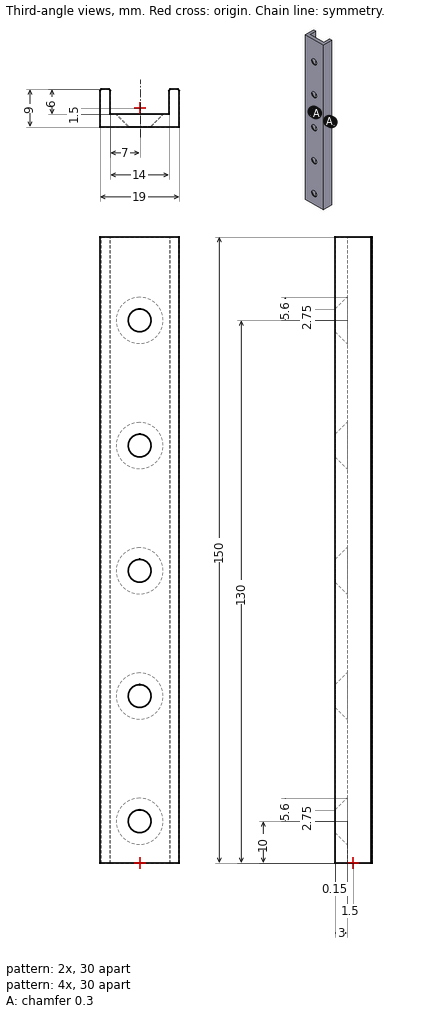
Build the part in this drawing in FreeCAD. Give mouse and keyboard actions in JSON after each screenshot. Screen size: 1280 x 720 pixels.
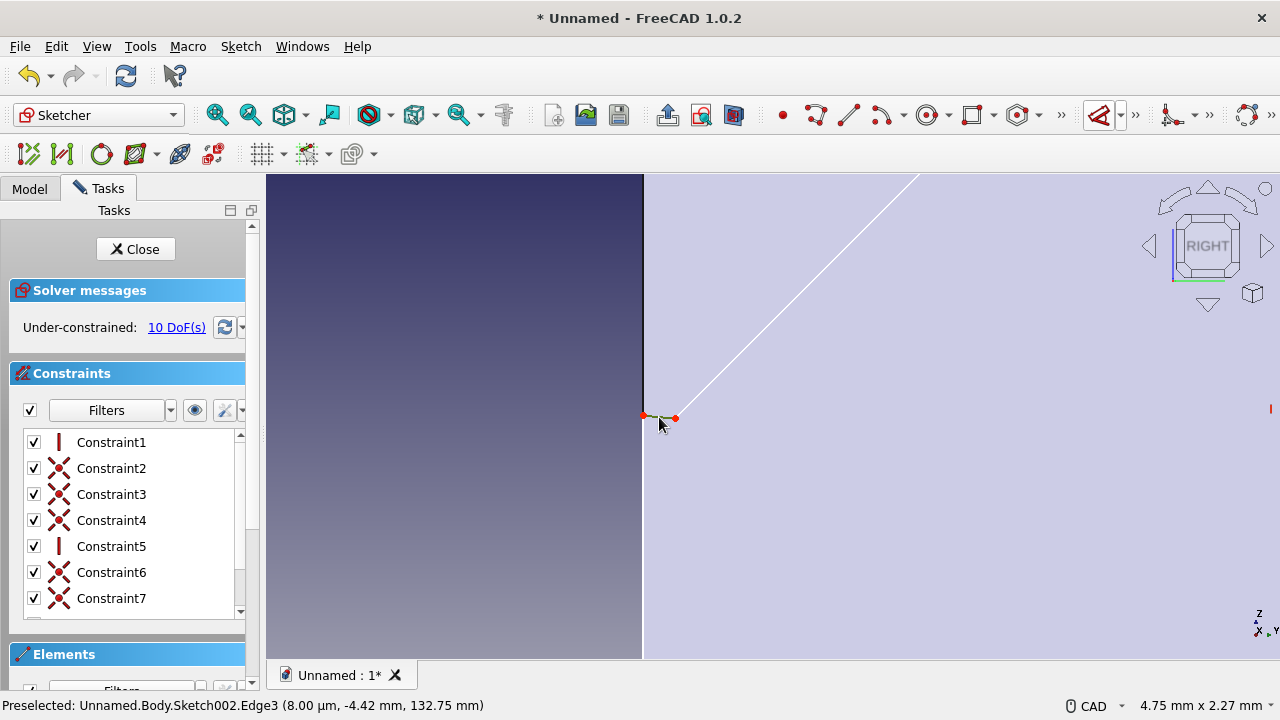
{"action": "key", "text": "h"}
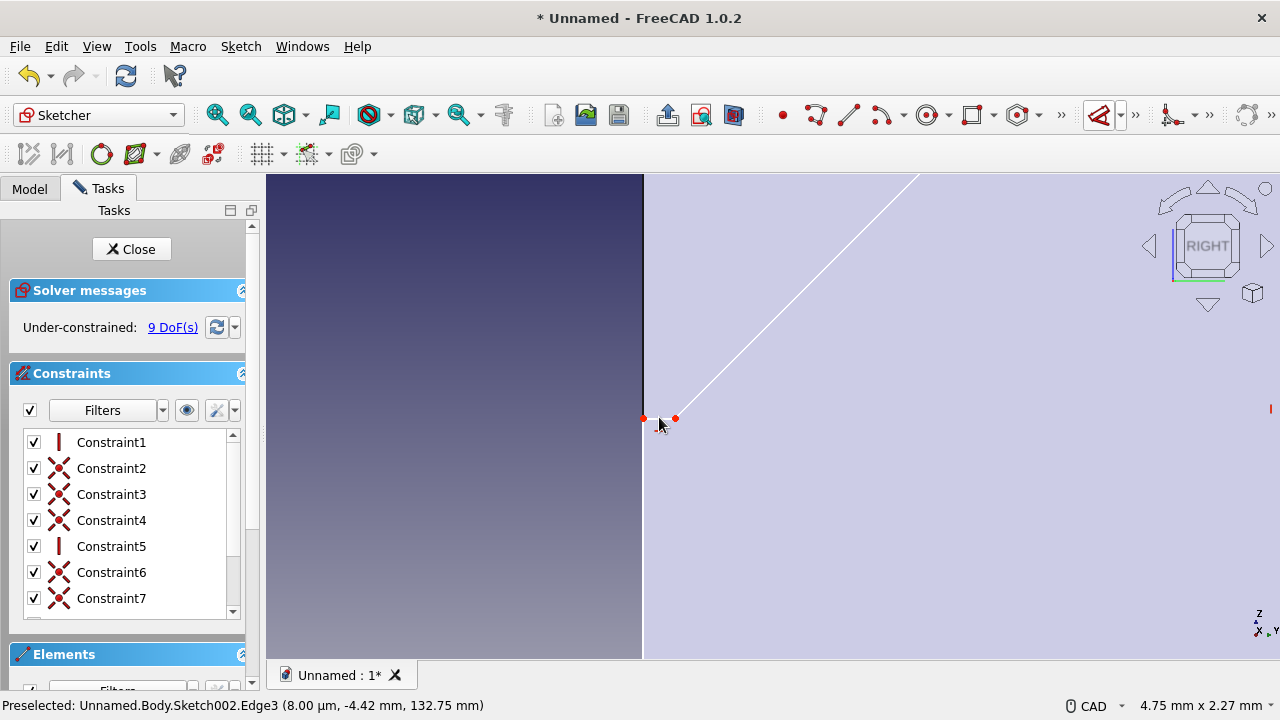
{"action": "scroll", "coordinate": [662, 420], "scroll_direction": "down", "scroll_amount": 7}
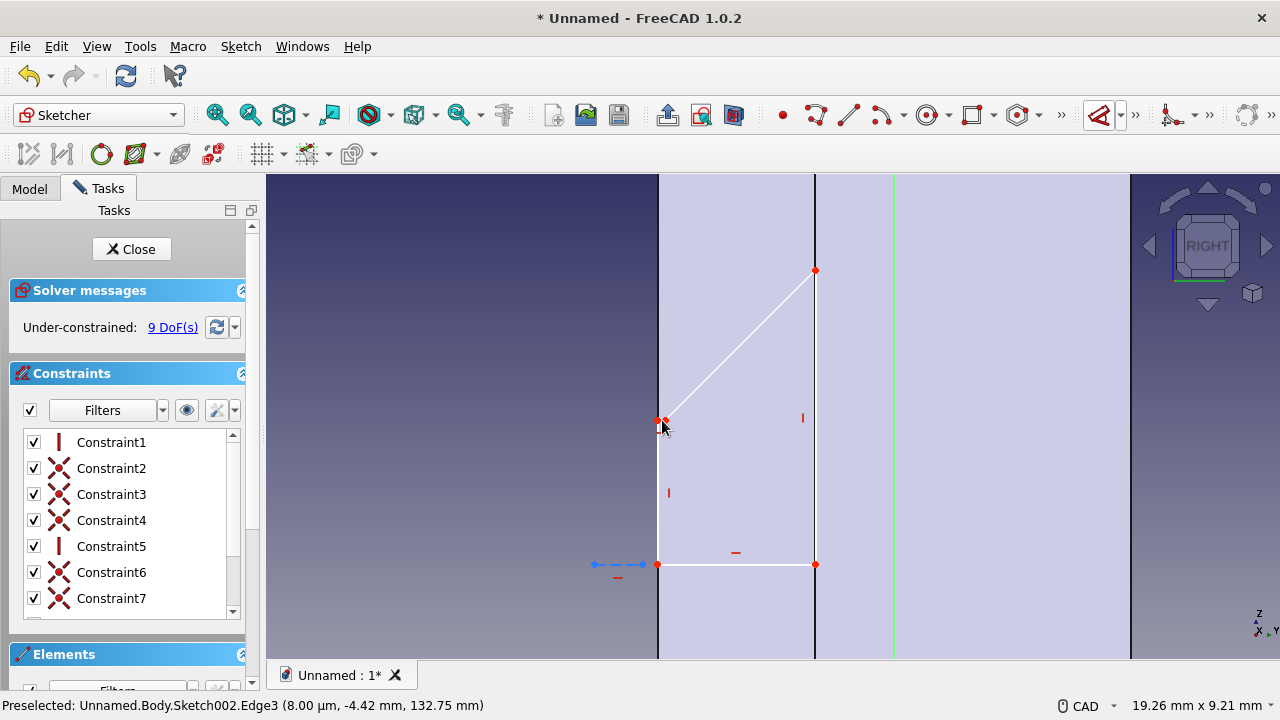
{"action": "left_click", "coordinate": [705, 565]}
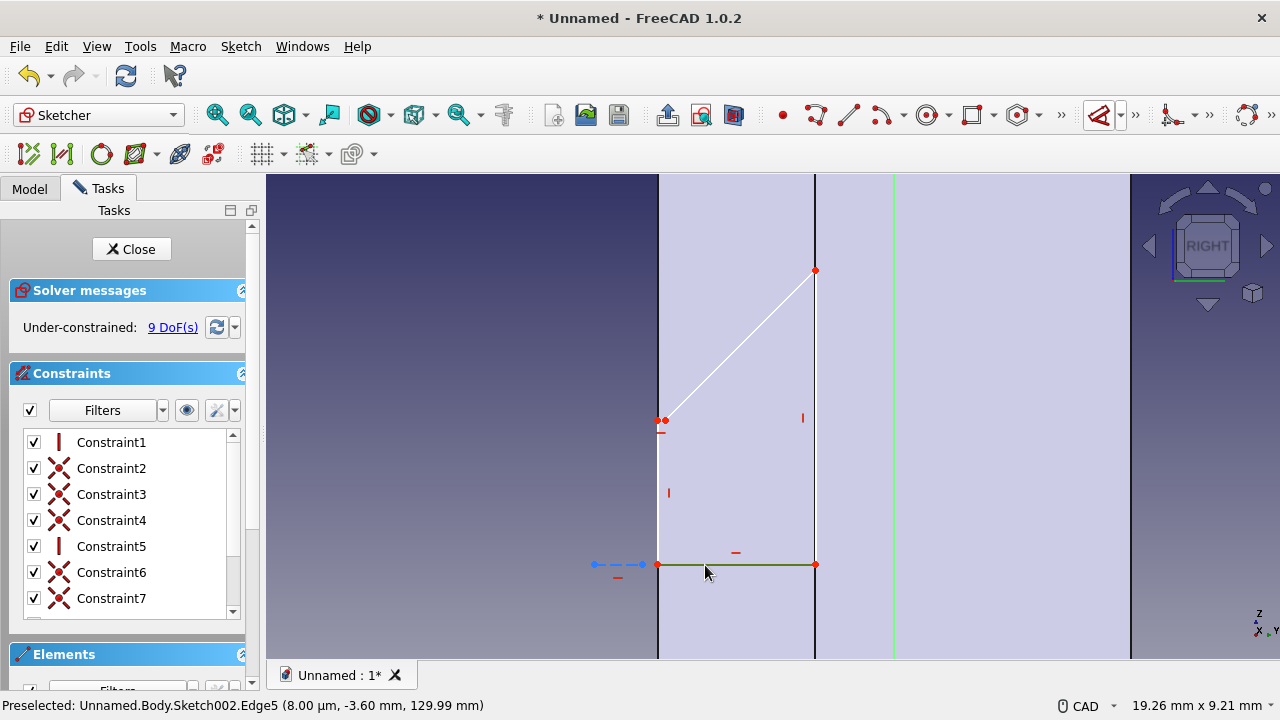
{"action": "left_click", "coordinate": [1120, 116]}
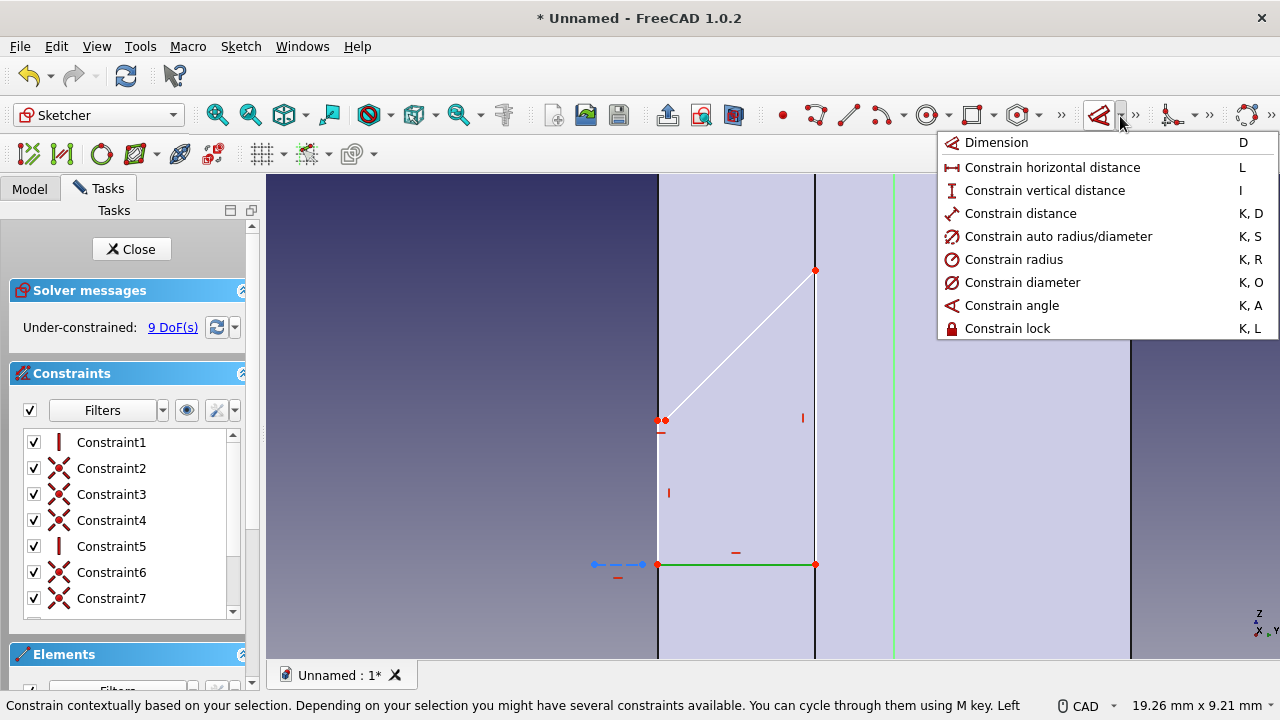
{"action": "left_click", "coordinate": [1108, 168]}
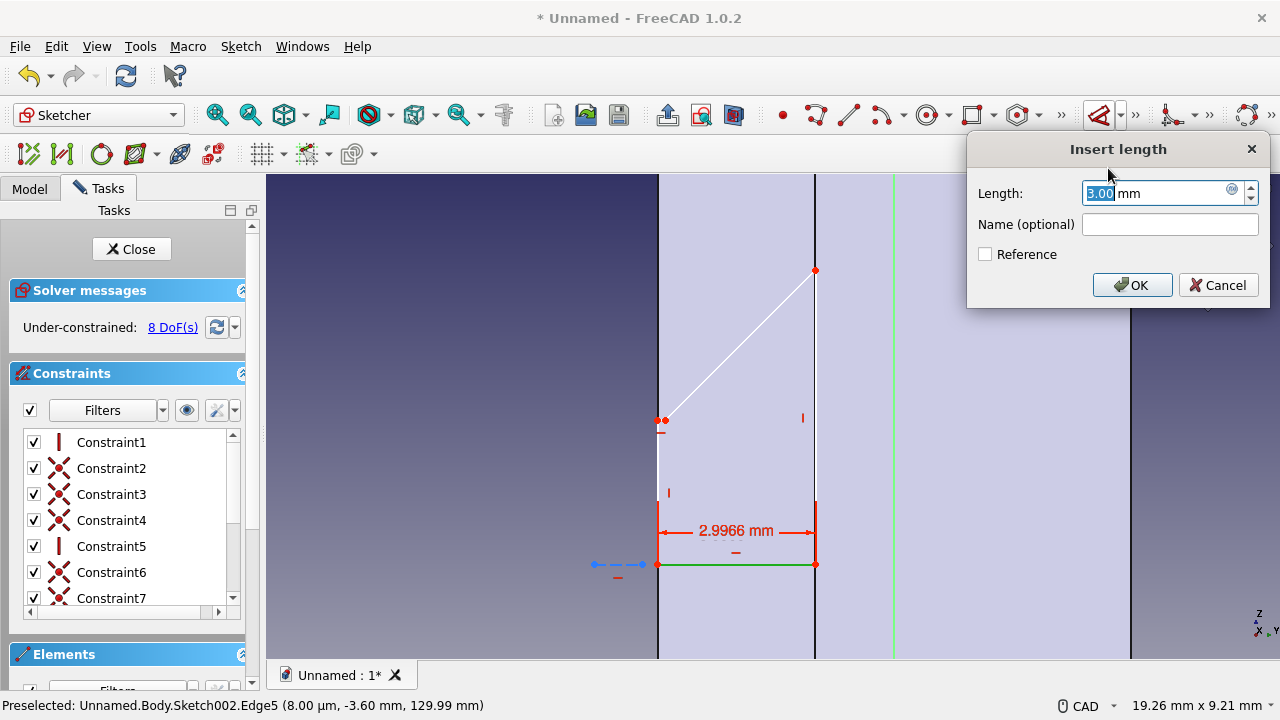
{"action": "type", "text": "3"}
{"action": "key", "text": "Return"}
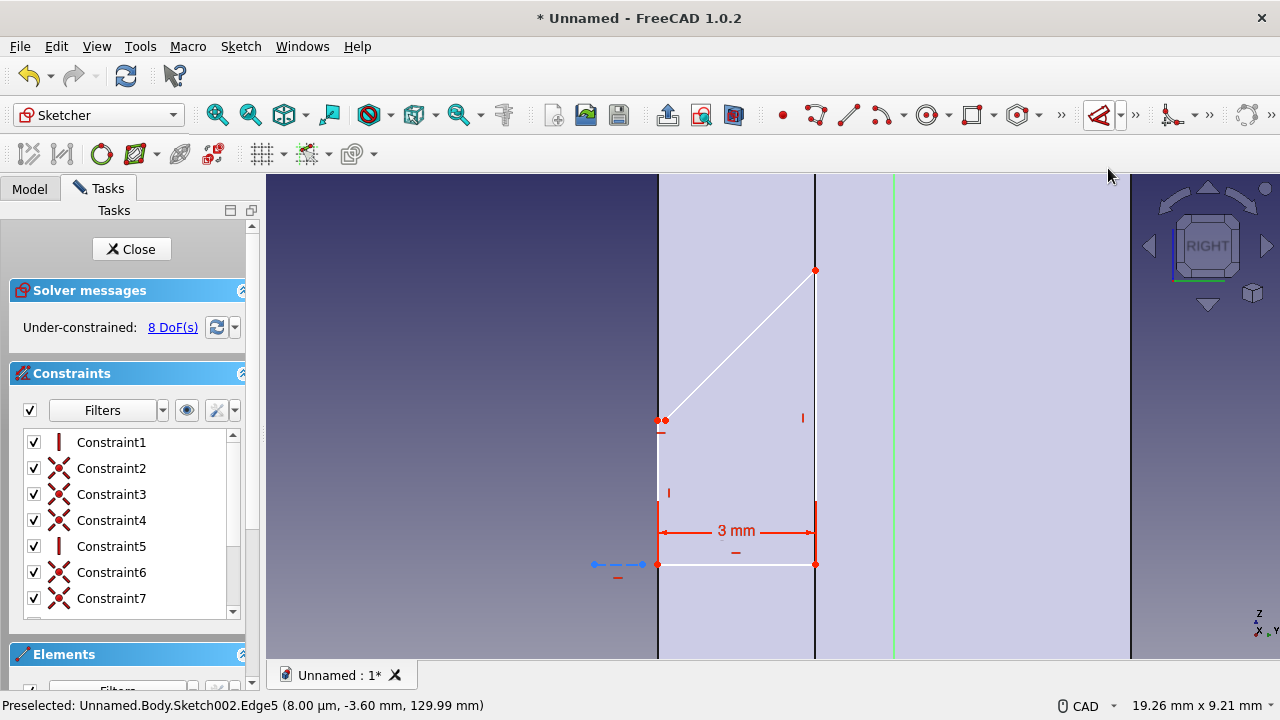
{"action": "left_click", "coordinate": [816, 477]}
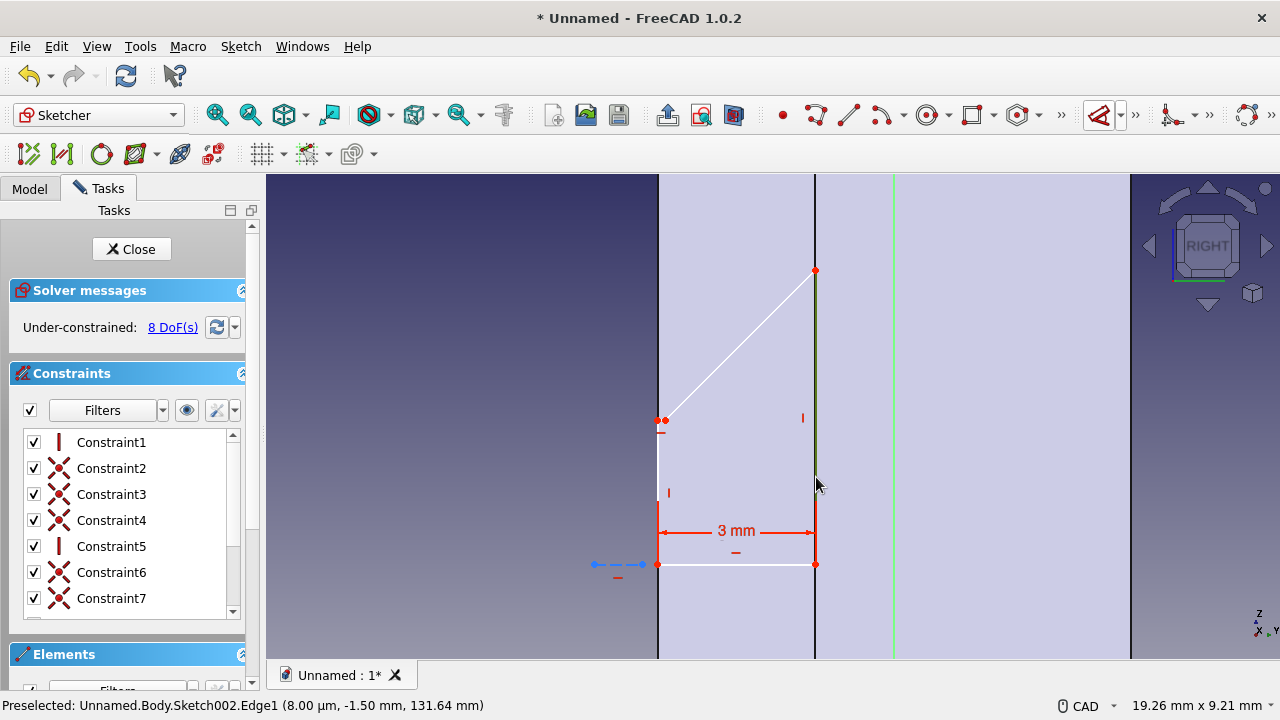
{"action": "left_click", "coordinate": [1120, 116]}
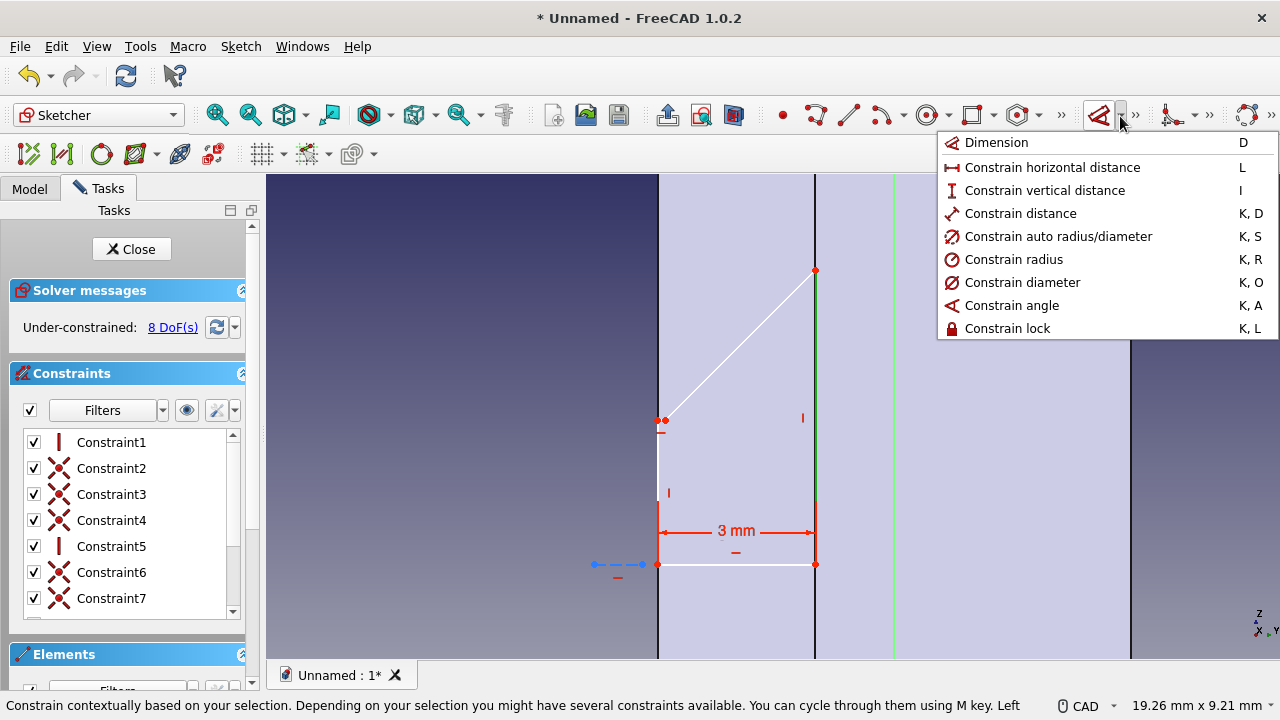
{"action": "left_click", "coordinate": [1108, 190]}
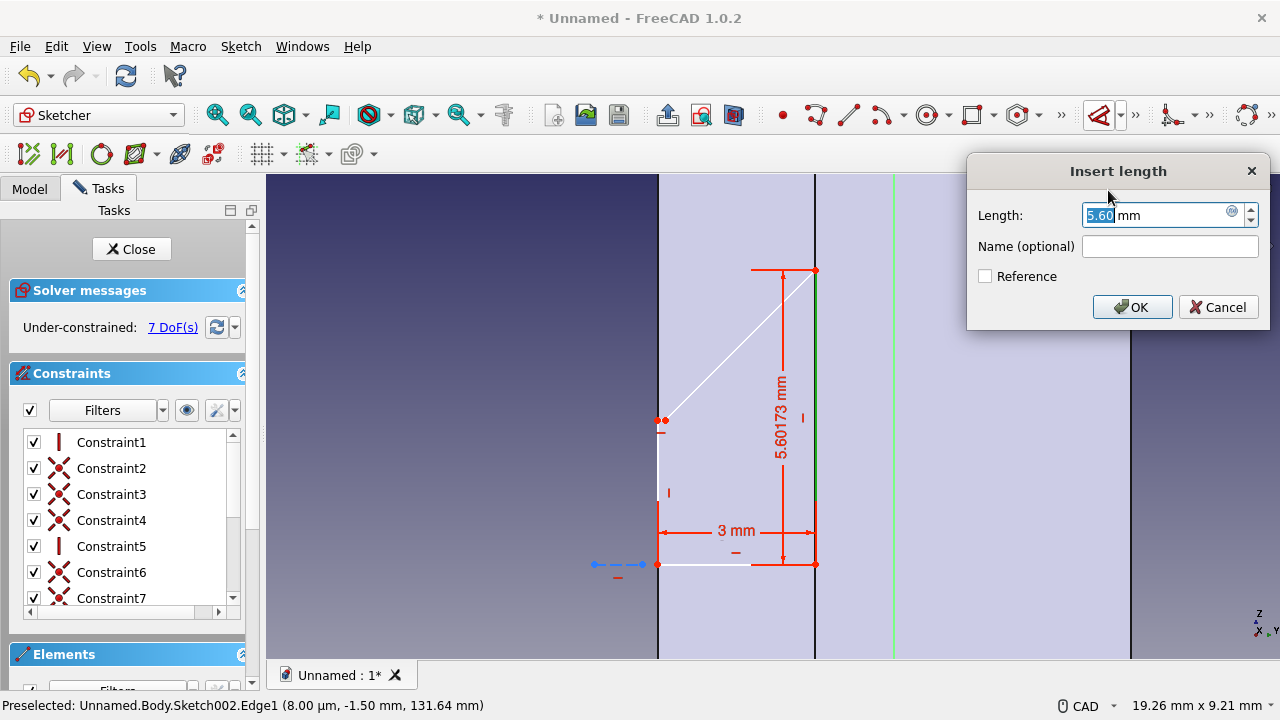
{"action": "type", "text": "5.6"}
{"action": "key", "text": "Return"}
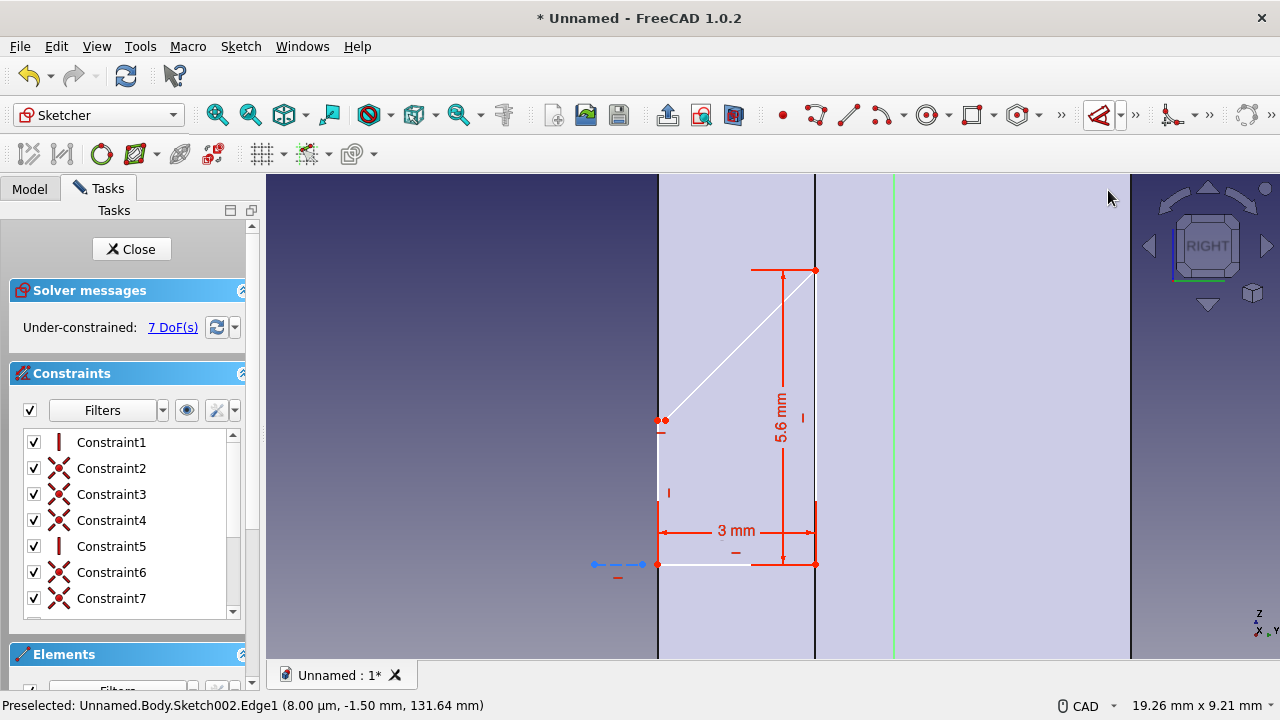
{"action": "scroll", "coordinate": [662, 420], "scroll_direction": "up", "scroll_amount": 9}